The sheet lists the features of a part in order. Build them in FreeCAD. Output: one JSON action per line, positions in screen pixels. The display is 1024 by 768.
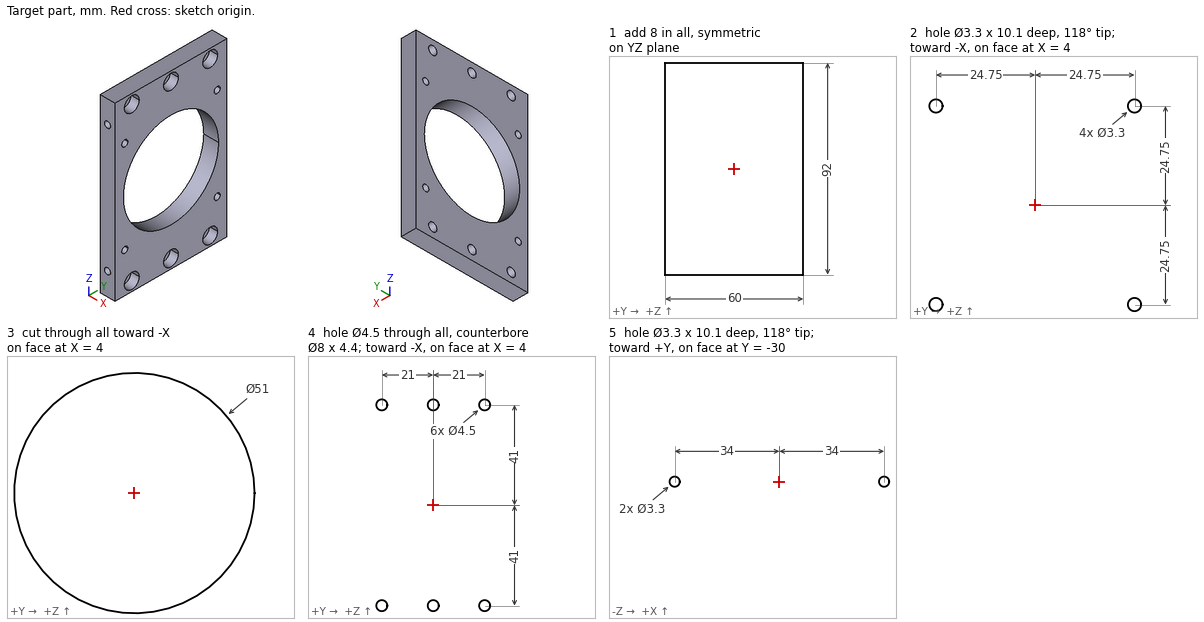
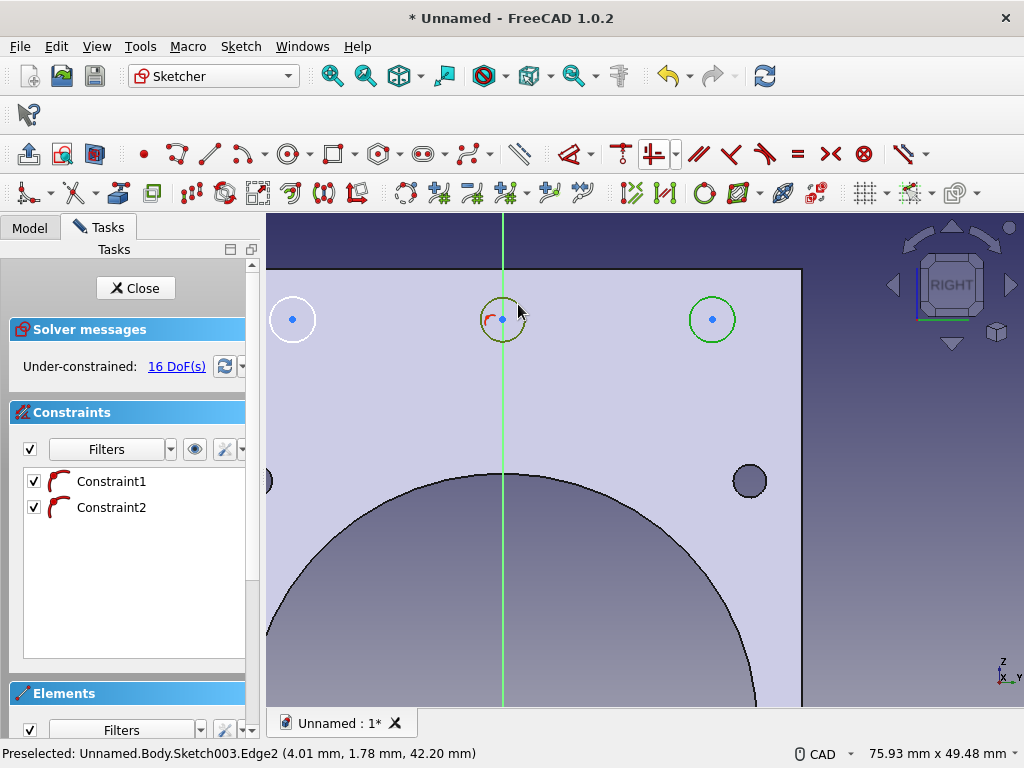
{"action": "left_click", "coordinate": [309, 304]}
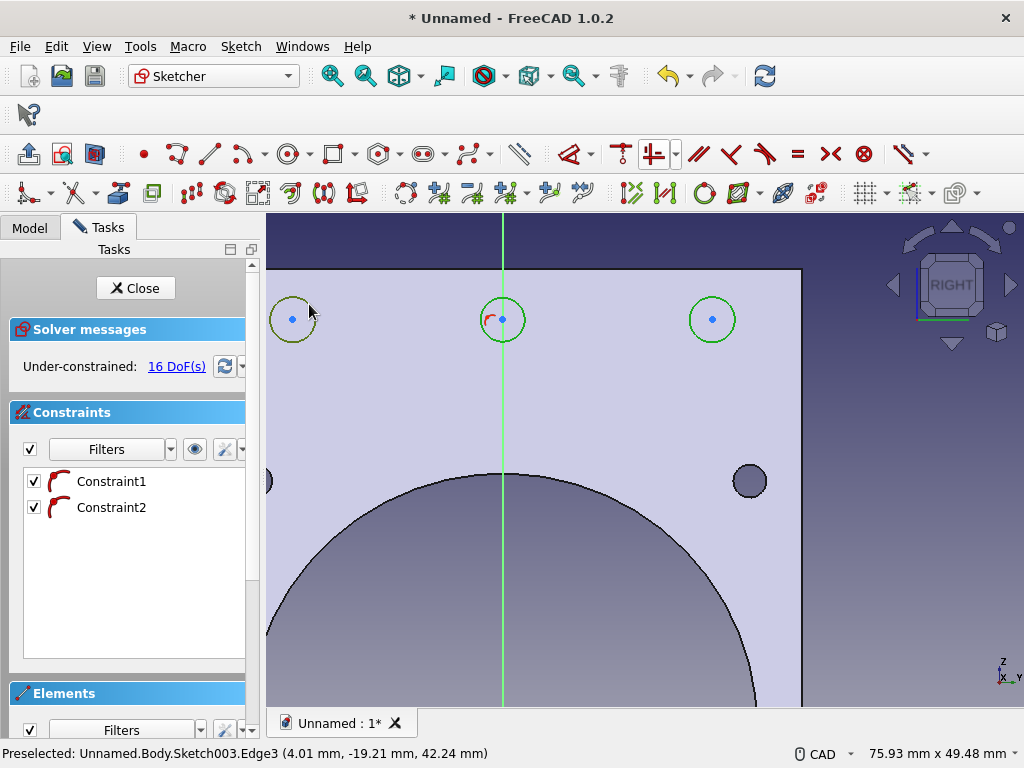
{"action": "scroll", "coordinate": [619, 304], "scroll_direction": "down", "scroll_amount": 5}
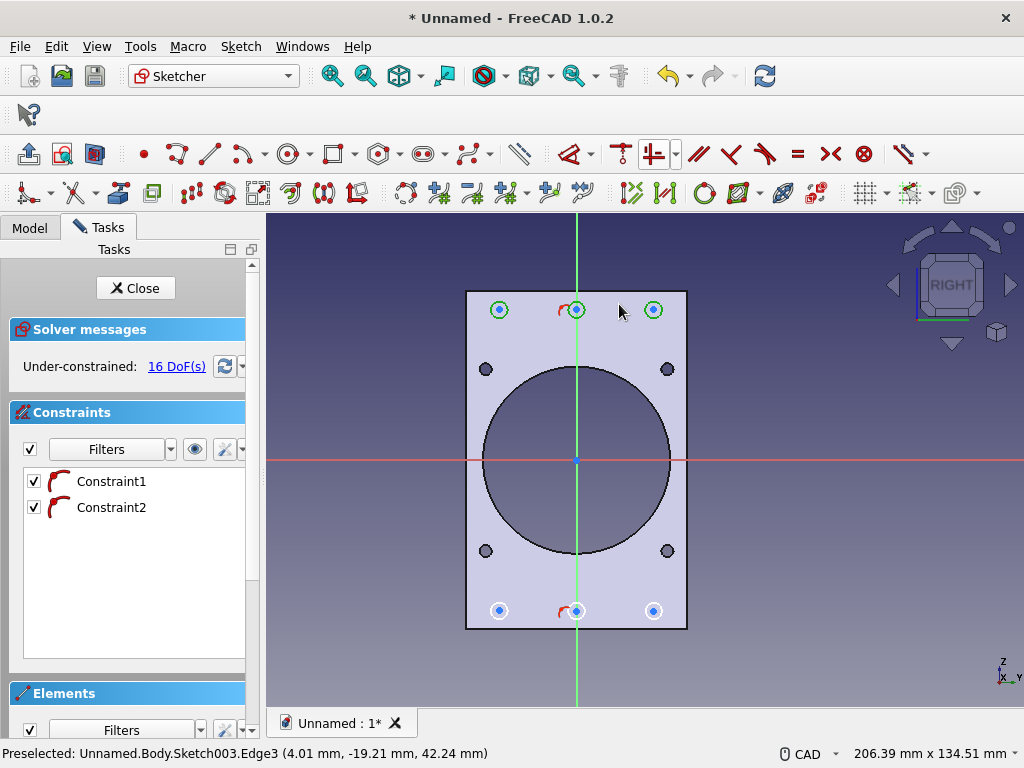
{"action": "scroll", "coordinate": [660, 605], "scroll_direction": "up", "scroll_amount": 3}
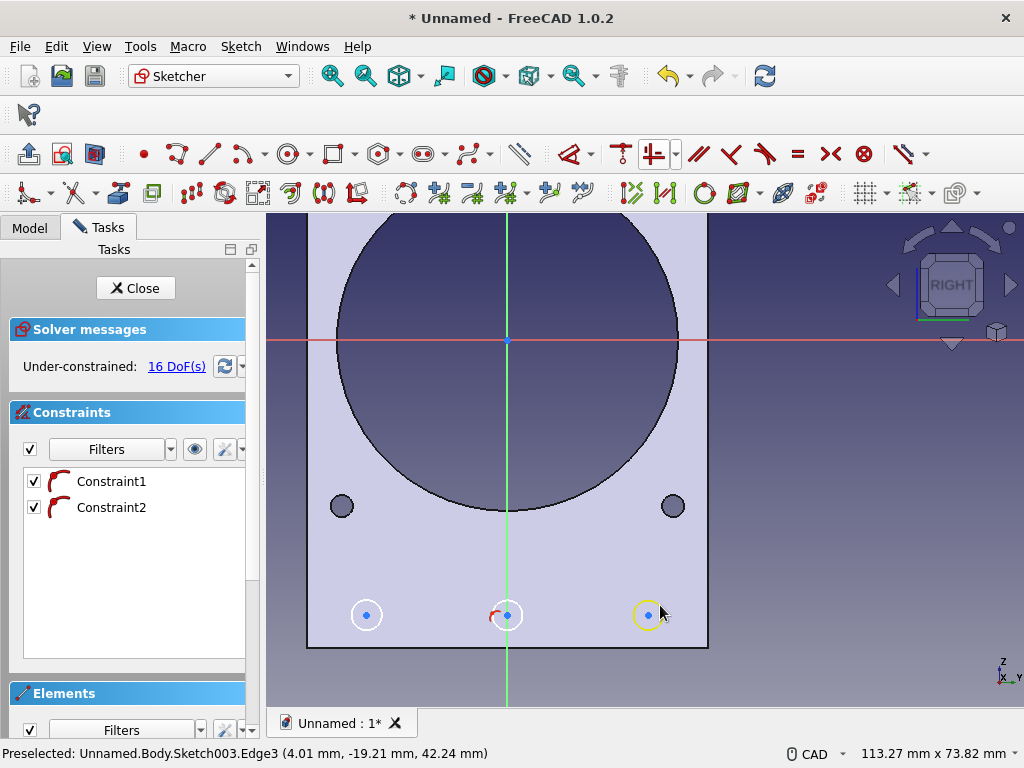
{"action": "left_click", "coordinate": [659, 605]}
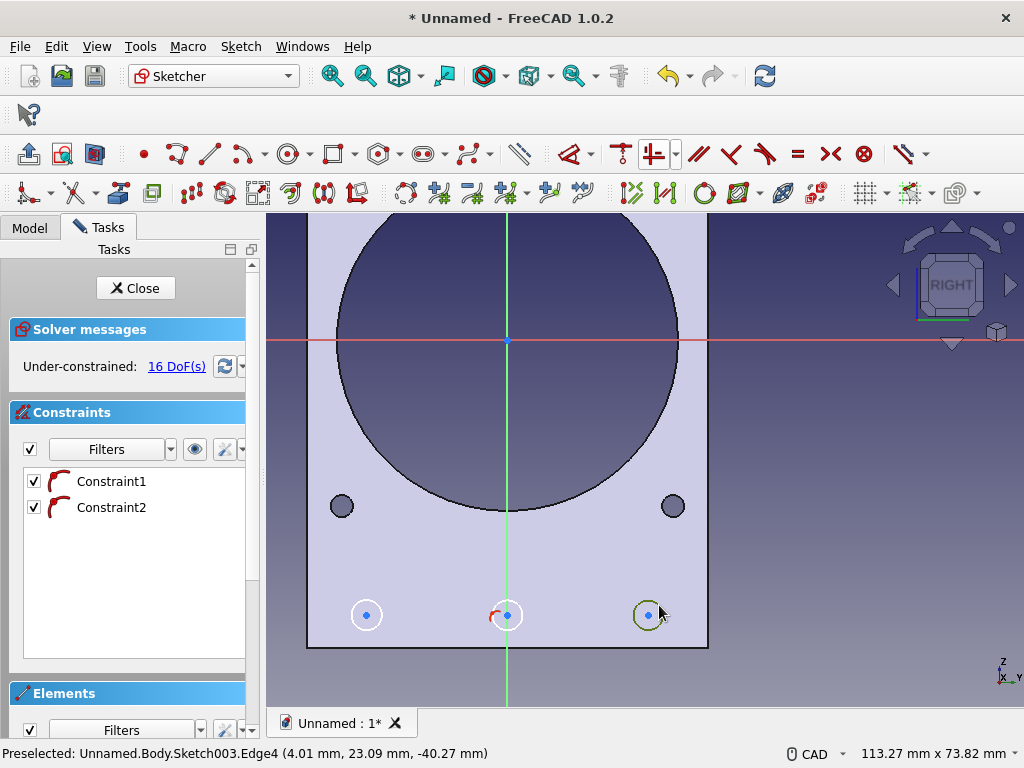
{"action": "scroll", "coordinate": [518, 605], "scroll_direction": "up", "scroll_amount": 2}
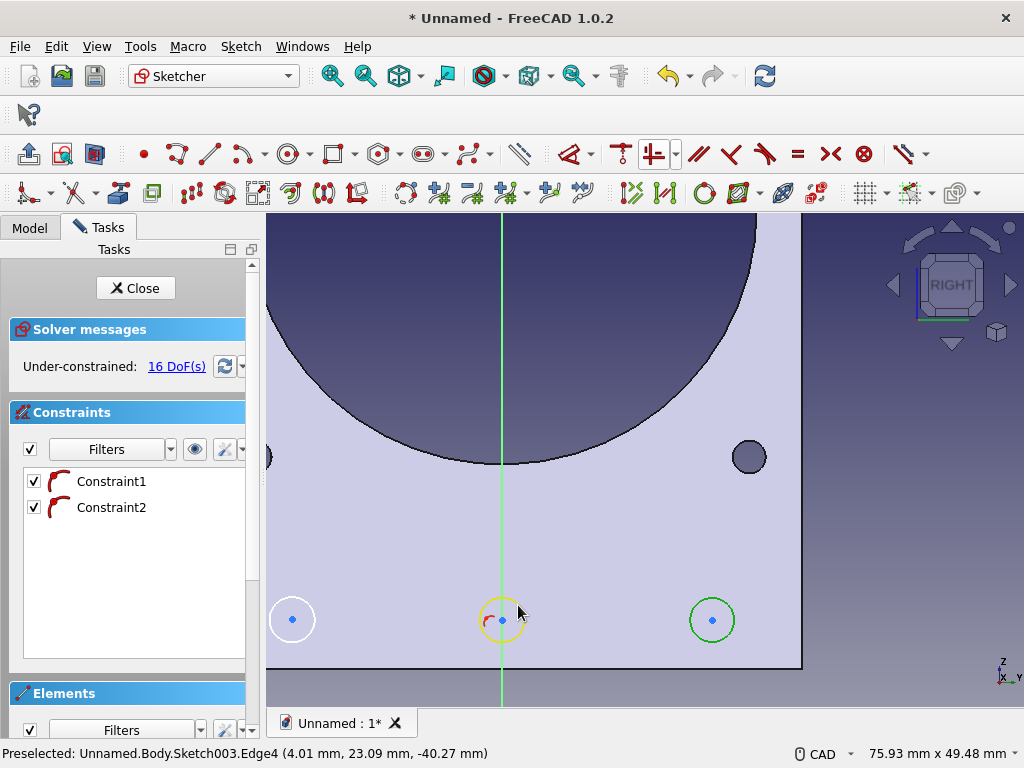
{"action": "left_click", "coordinate": [518, 604]}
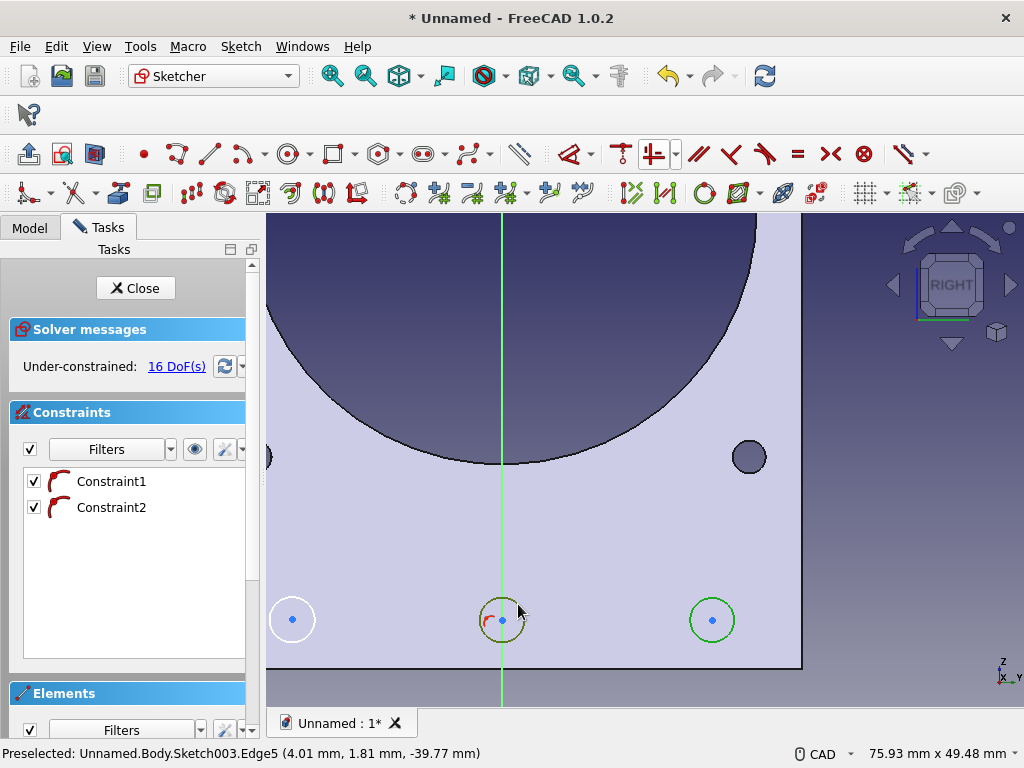
{"action": "left_click", "coordinate": [308, 604]}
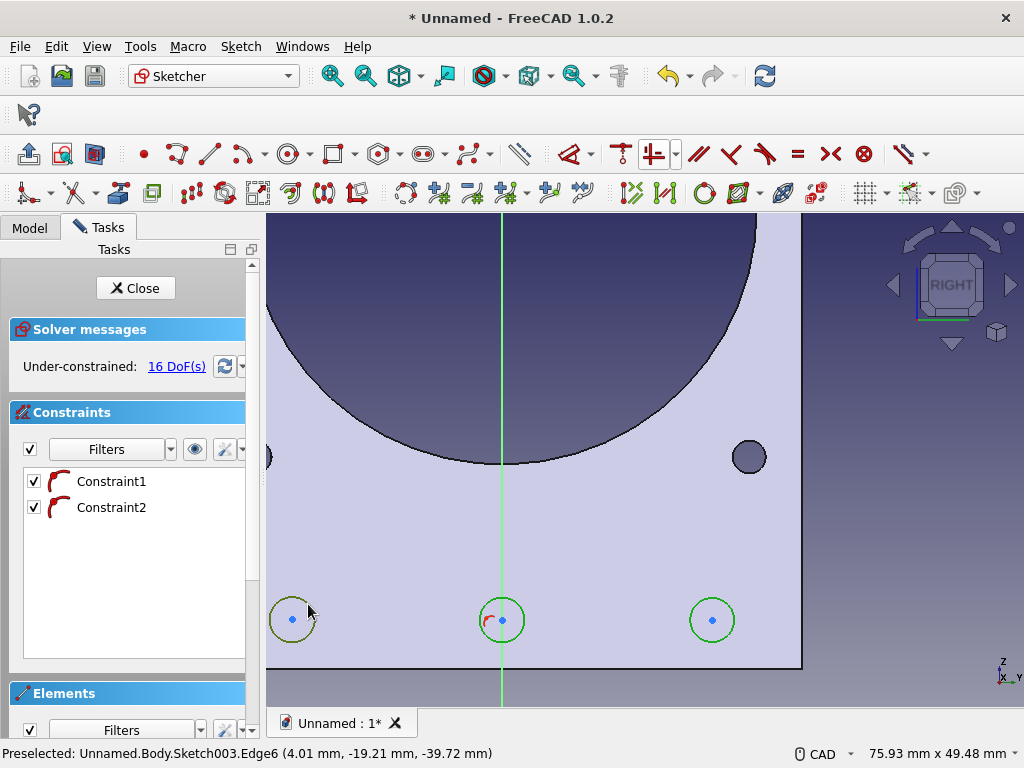
{"action": "left_click", "coordinate": [798, 154]}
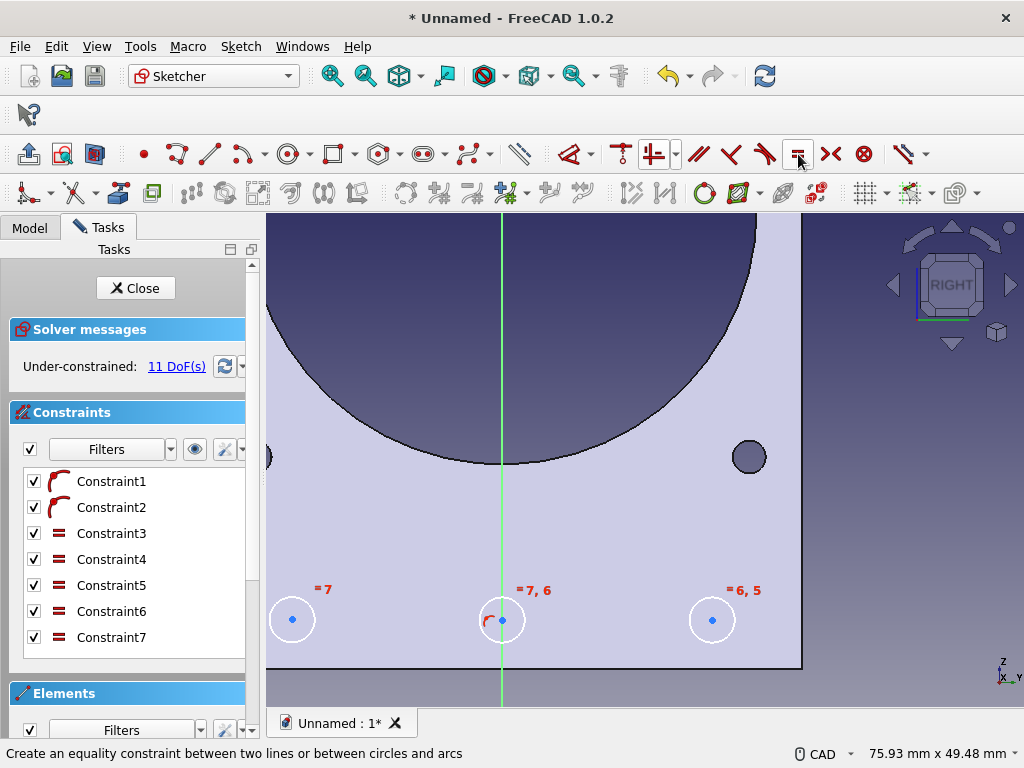
{"action": "scroll", "coordinate": [620, 606], "scroll_direction": "down", "scroll_amount": 5}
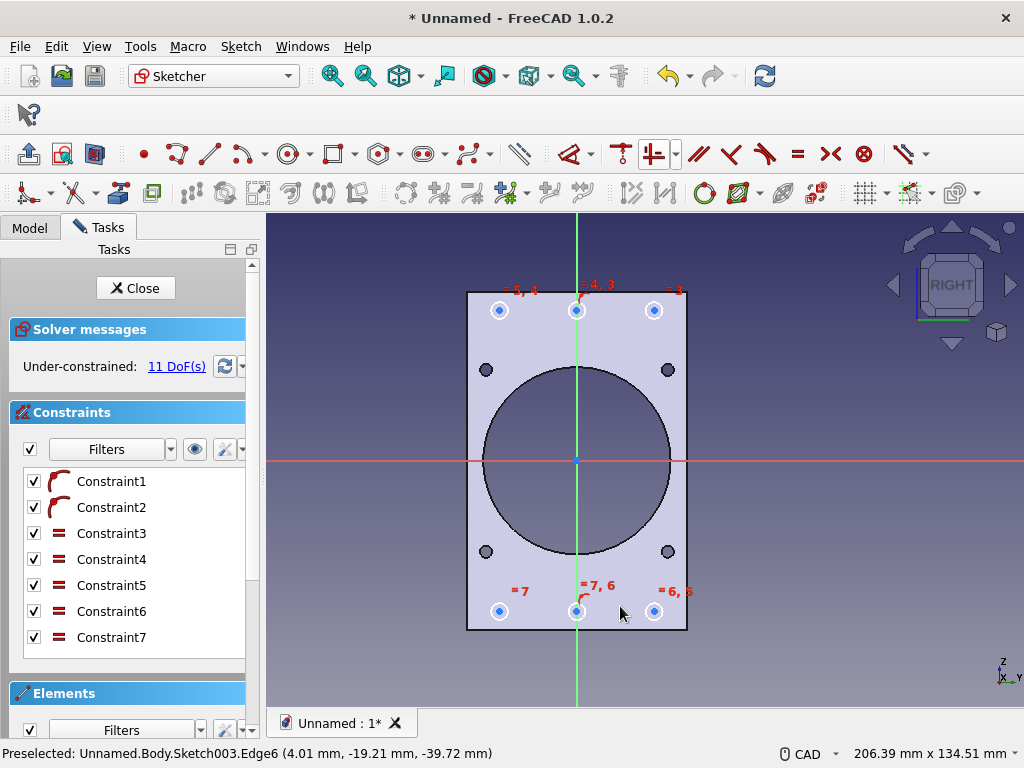
{"action": "left_click", "coordinate": [654, 311]}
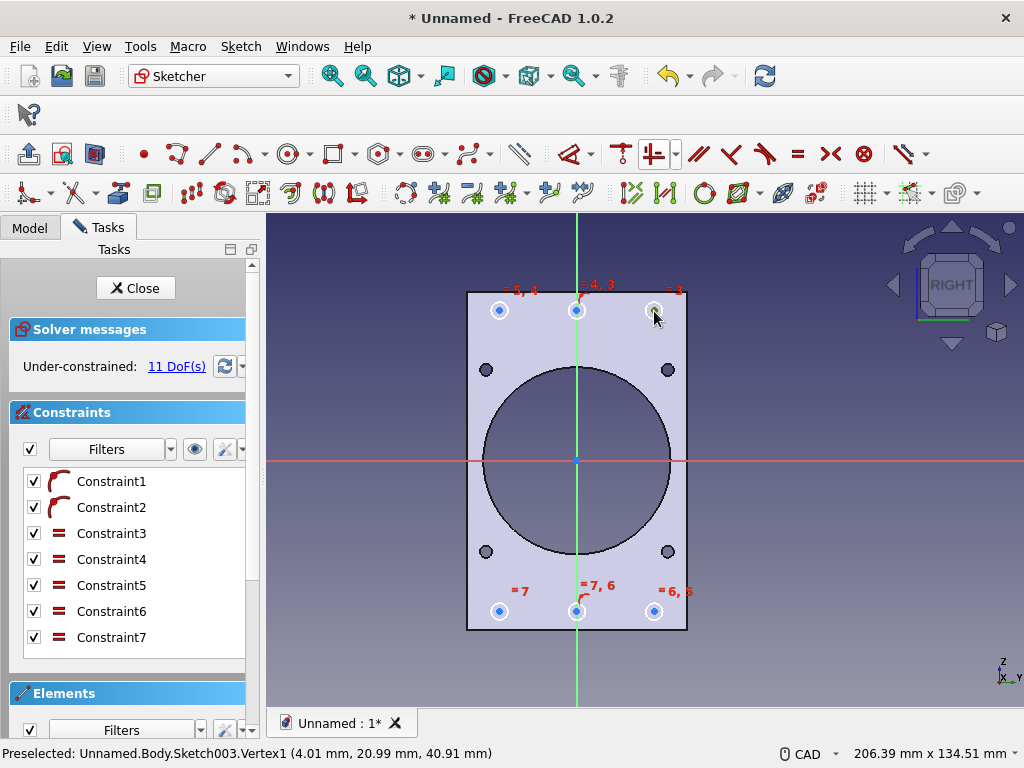
{"action": "left_click", "coordinate": [577, 311]}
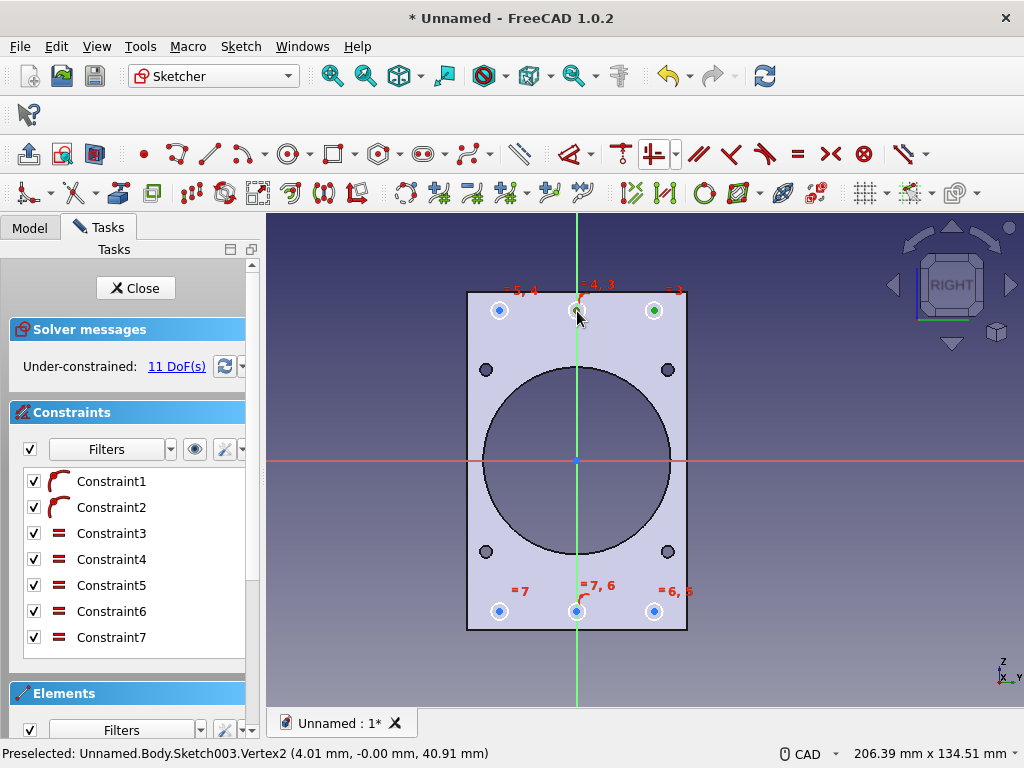
{"action": "left_click", "coordinate": [676, 154]}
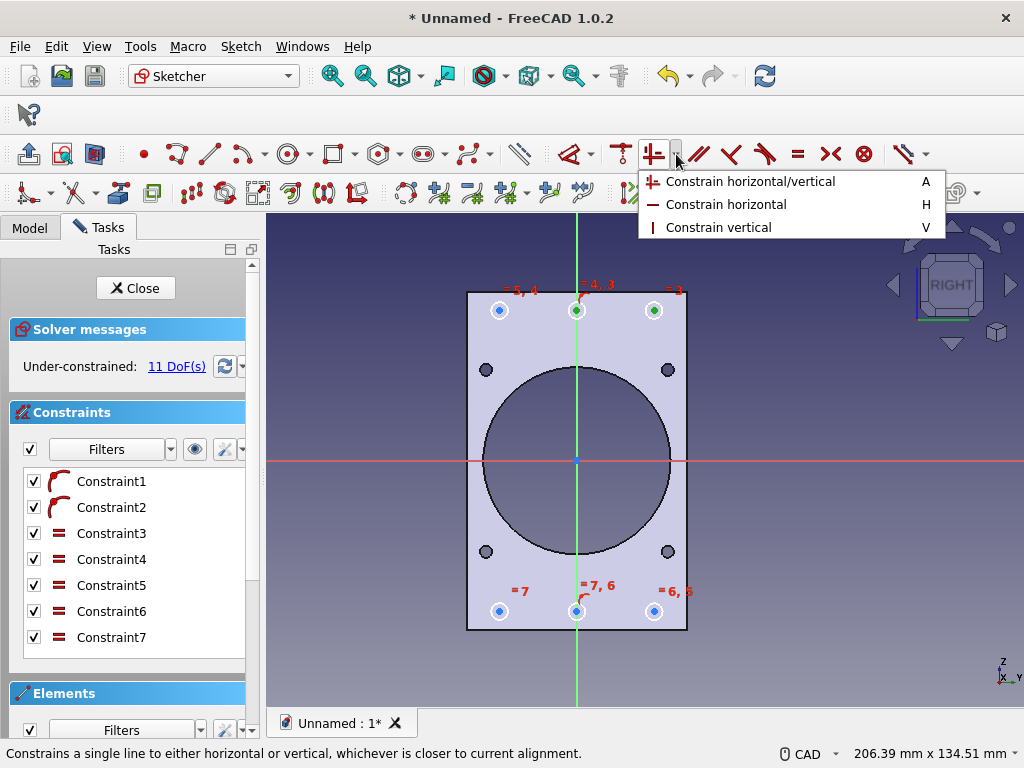
{"action": "left_click", "coordinate": [792, 204]}